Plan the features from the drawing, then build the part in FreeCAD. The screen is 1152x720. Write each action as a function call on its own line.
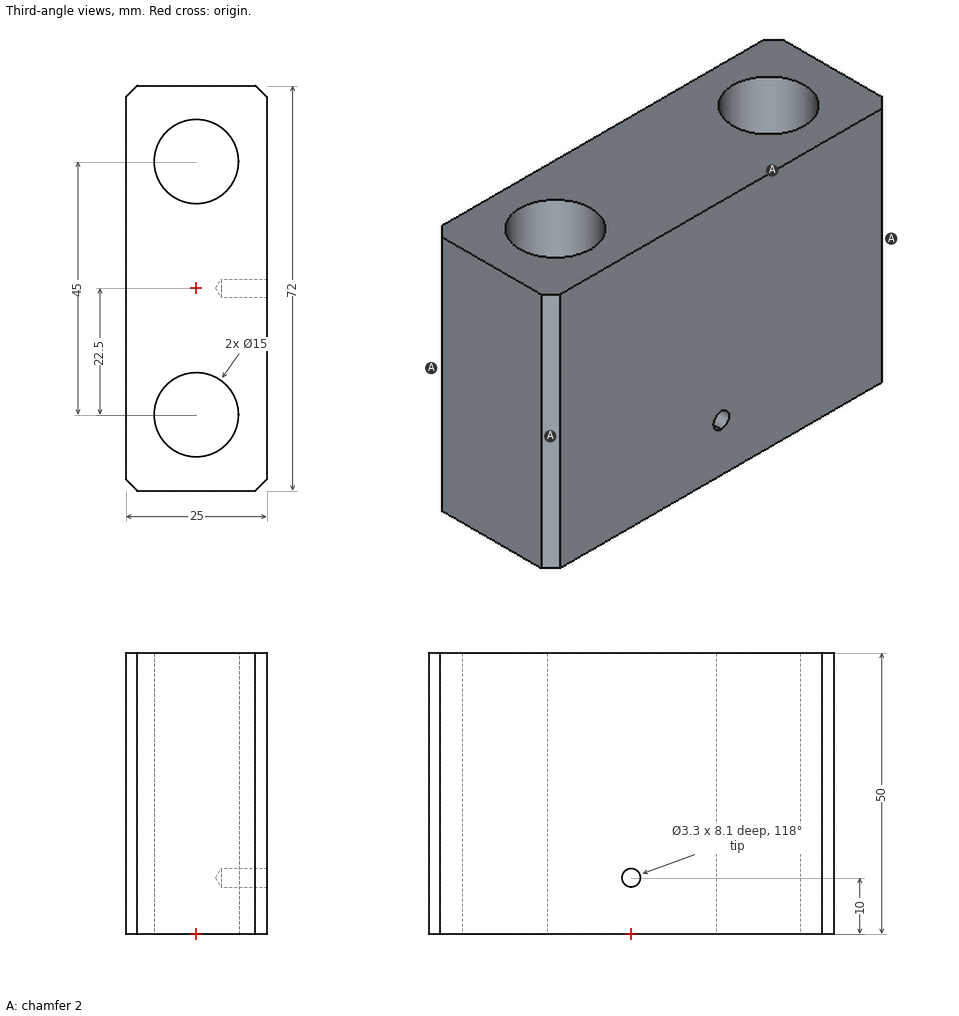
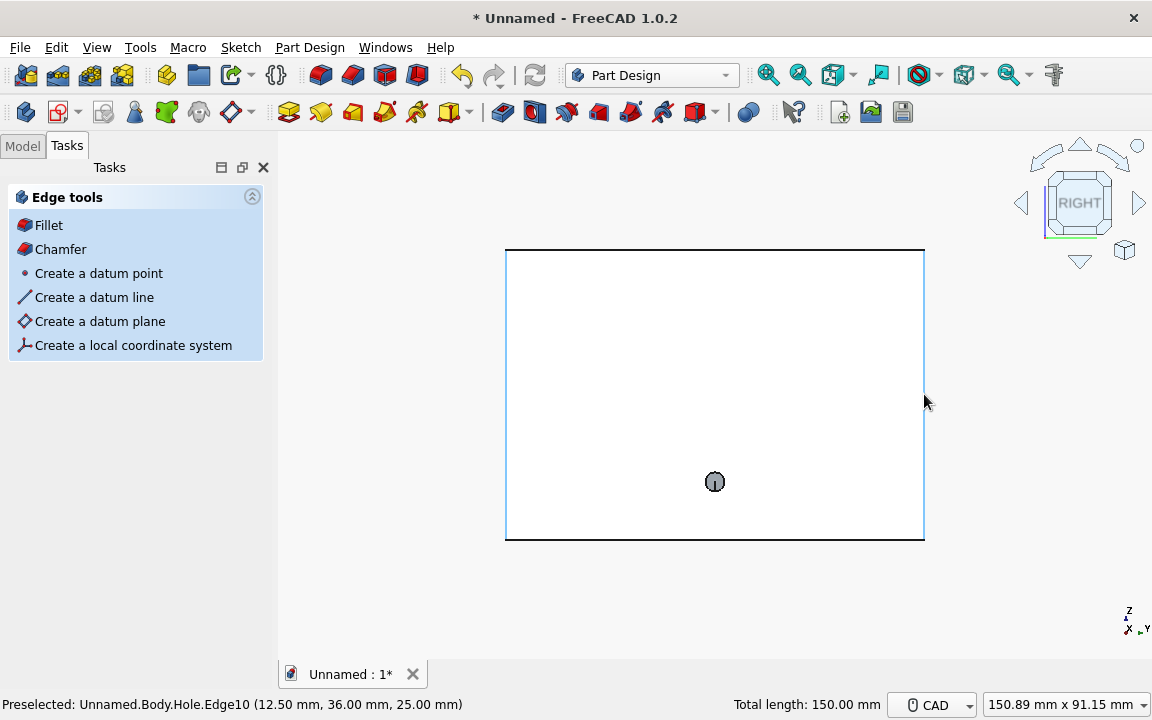
key(5)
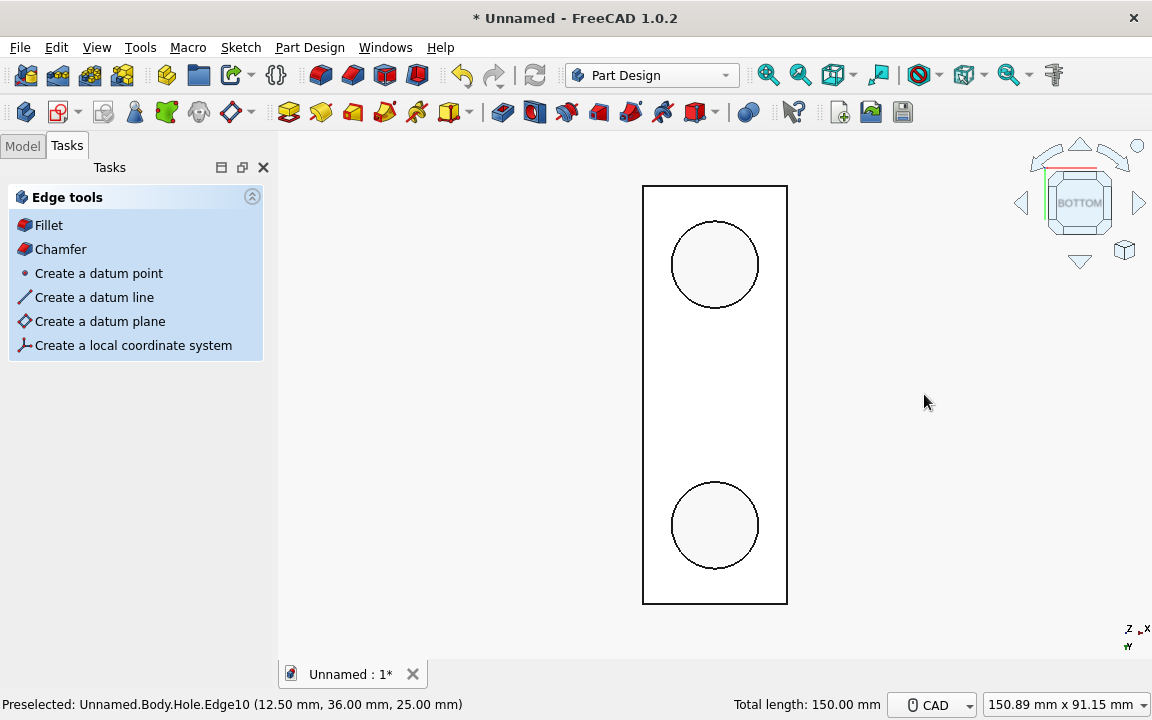
key(4)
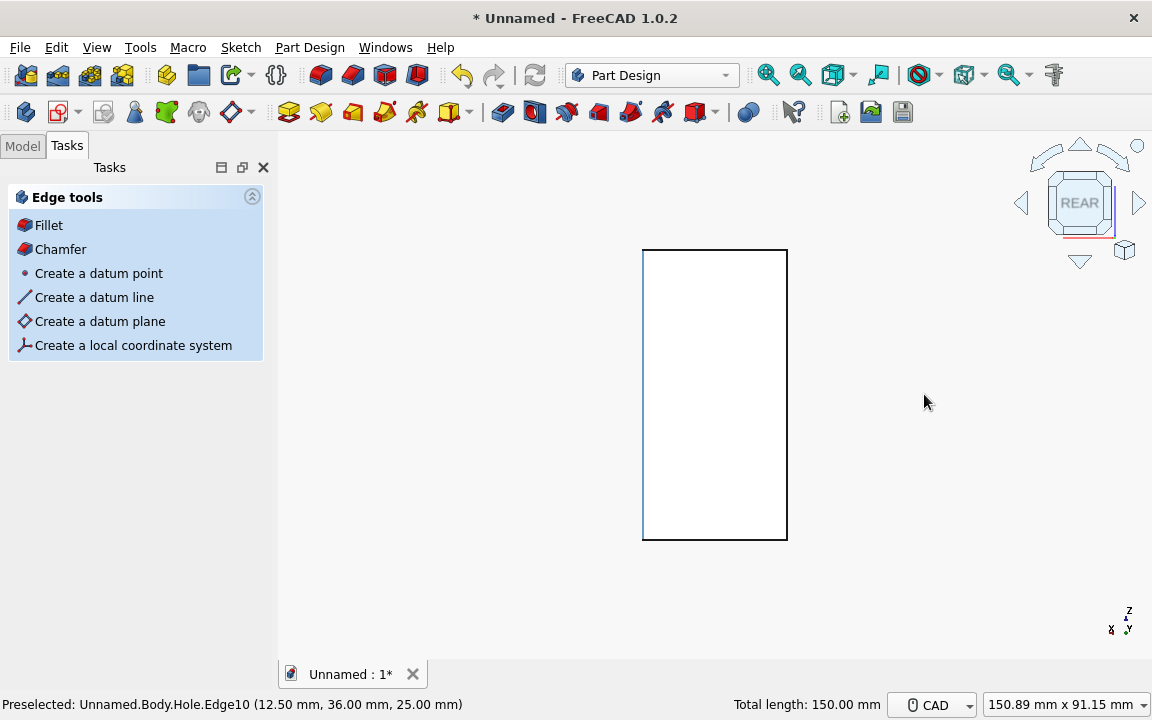
click(787, 394, ctrl)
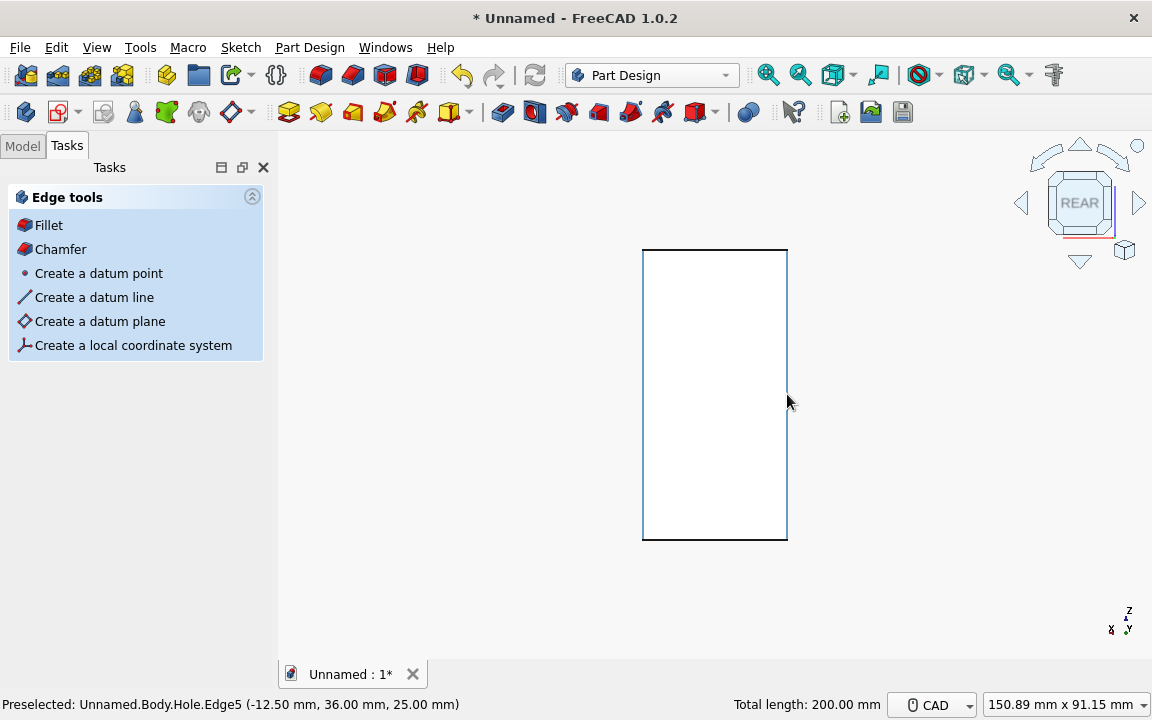
click(354, 76)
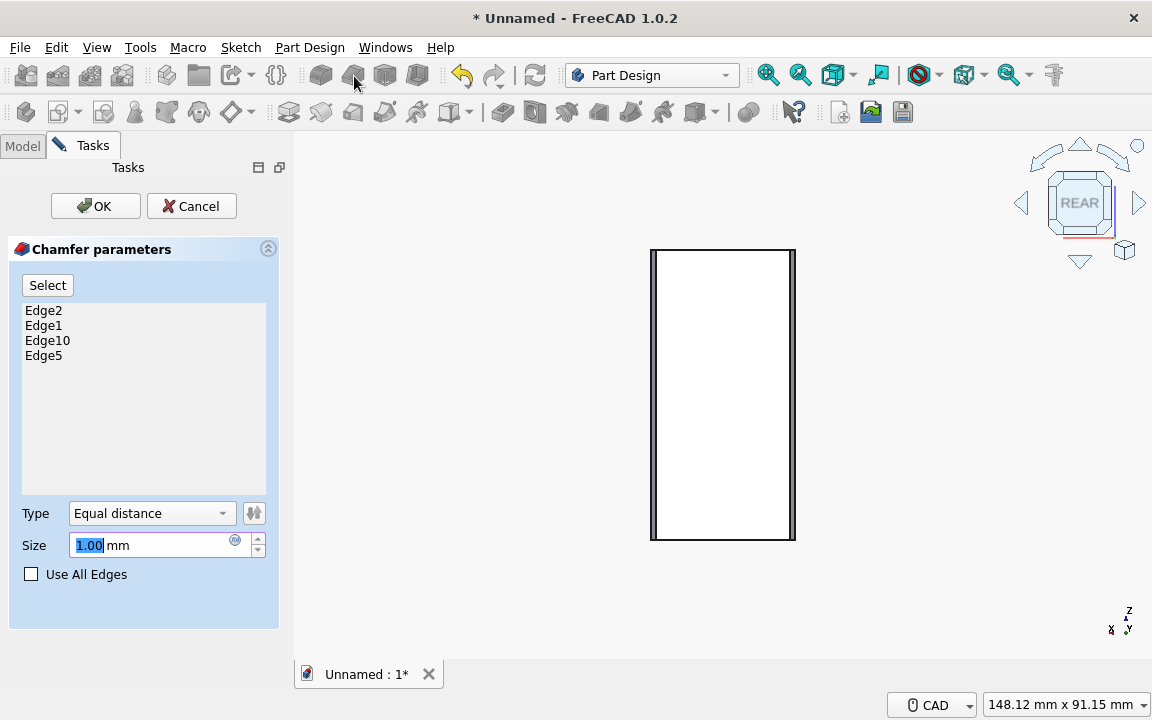
text(2)
key(Tab)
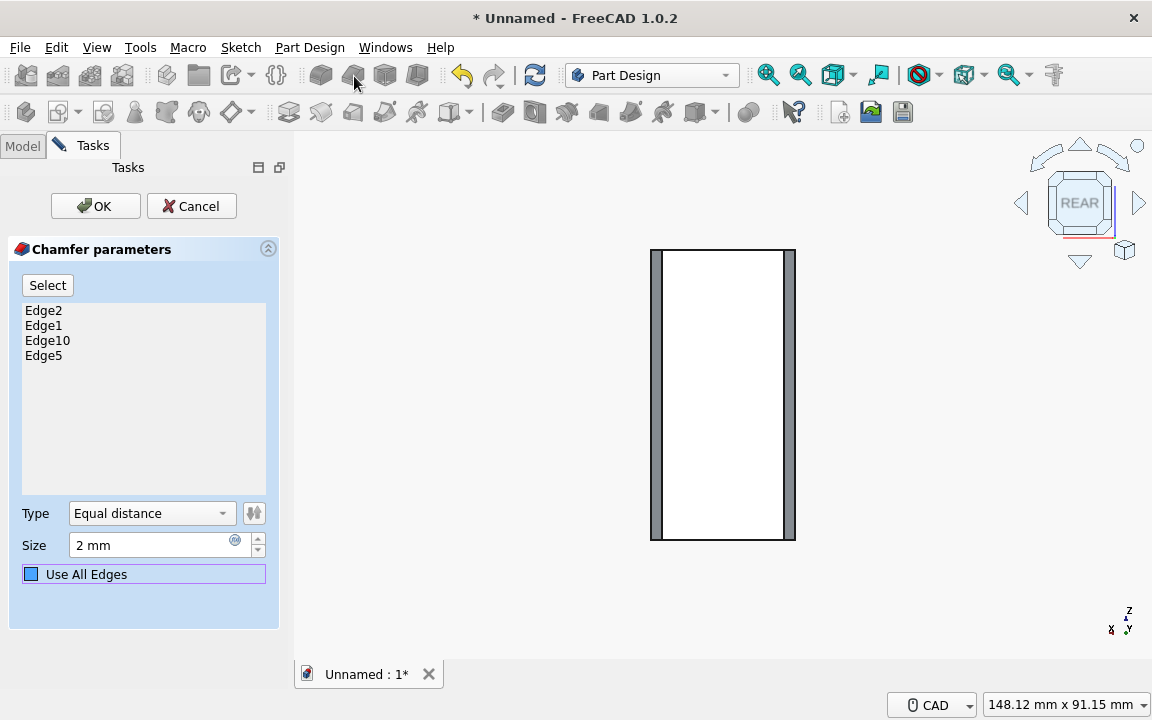
click(96, 206)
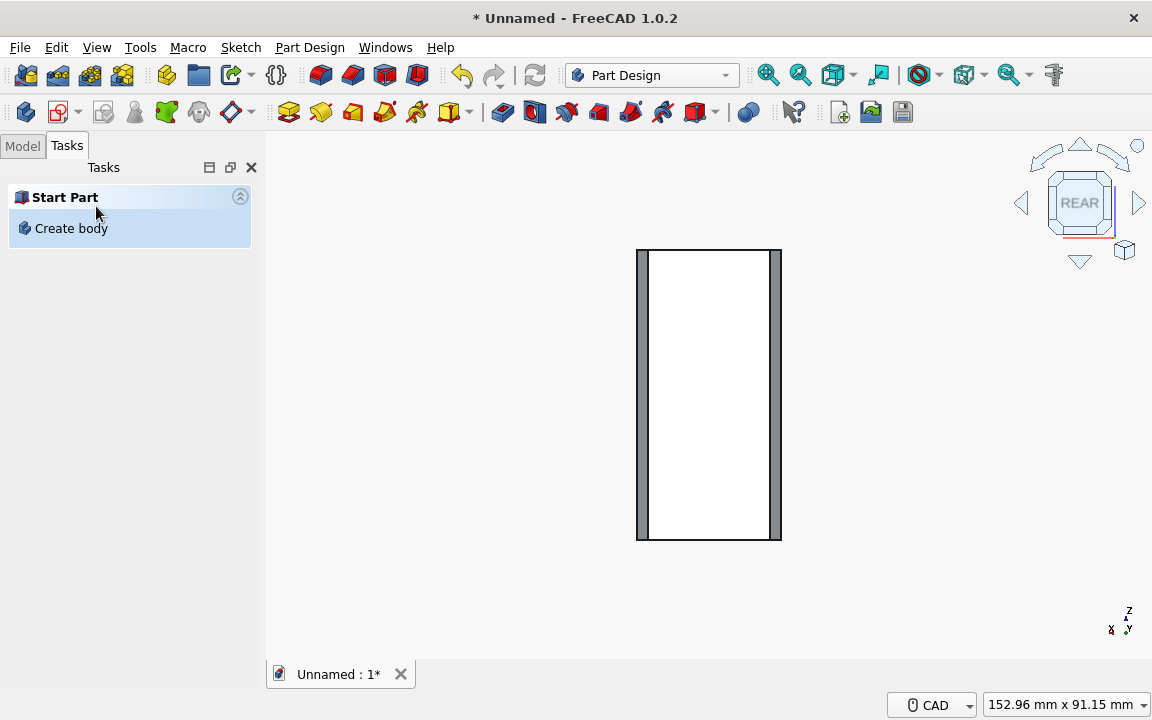
key(0)